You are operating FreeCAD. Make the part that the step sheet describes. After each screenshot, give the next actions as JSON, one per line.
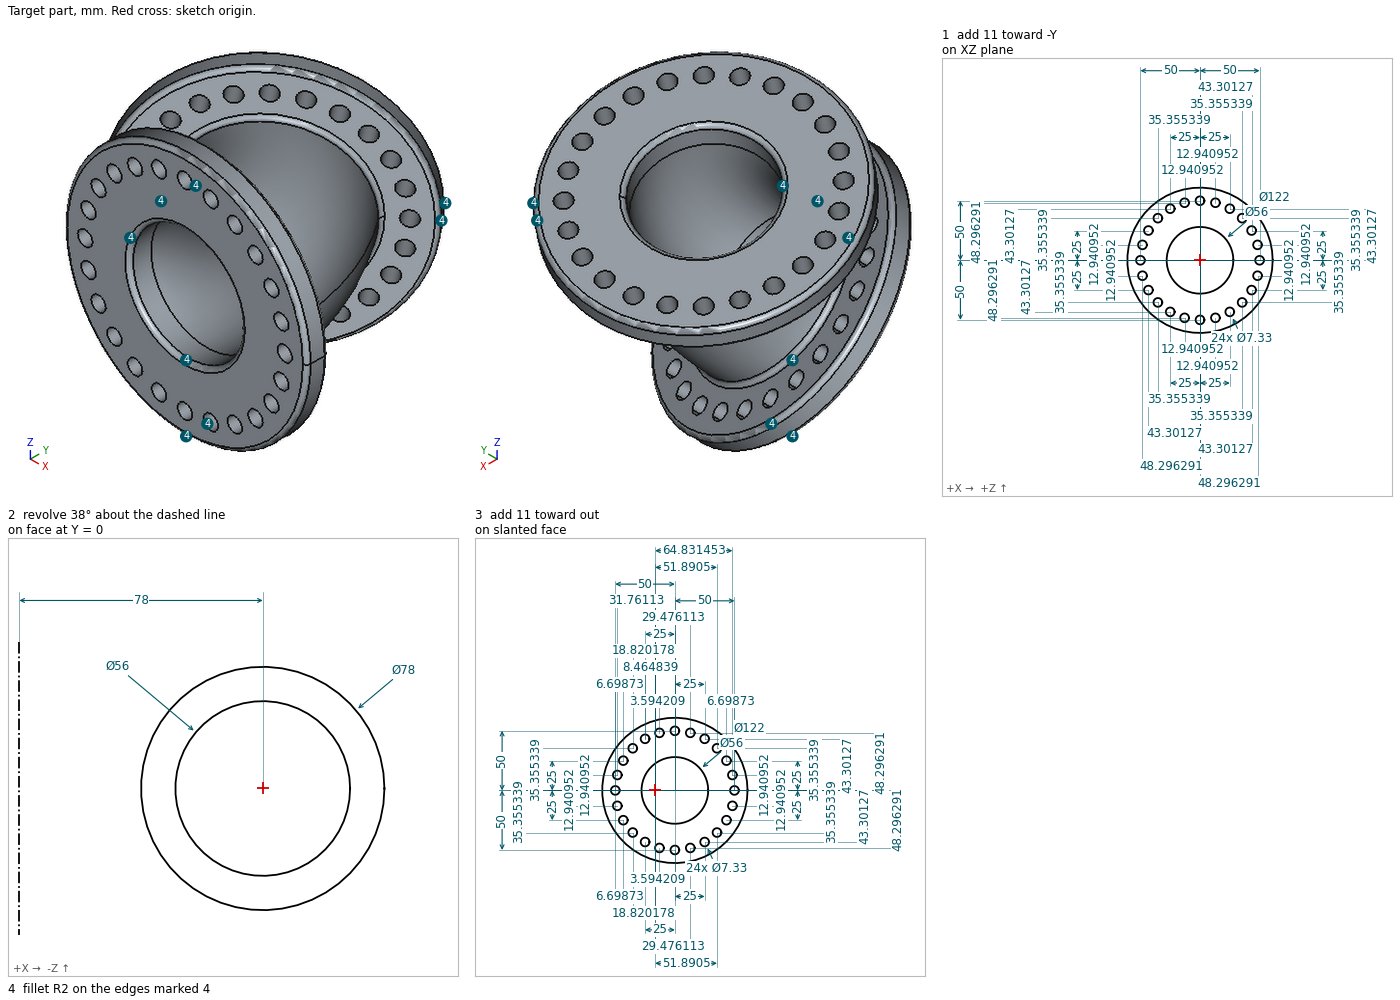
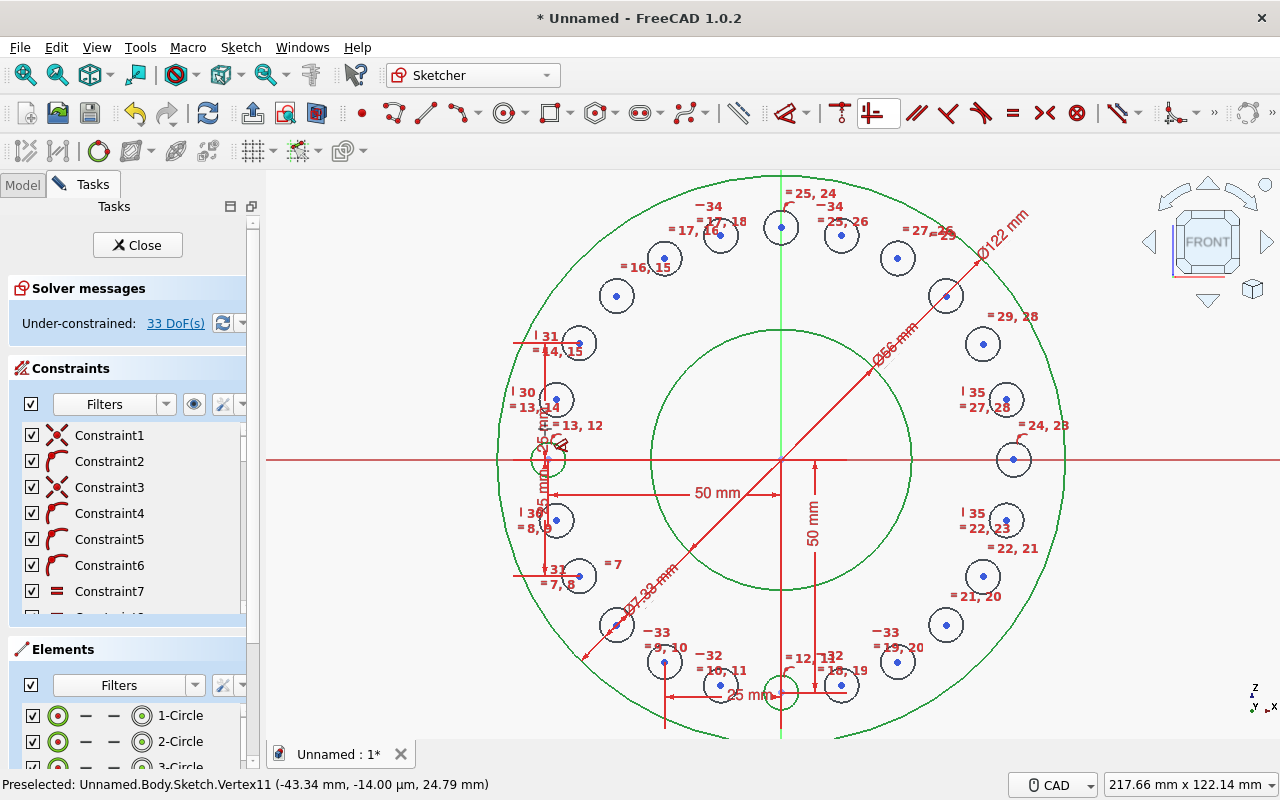
{"action": "left_click", "coordinate": [665, 259]}
{"action": "left_click", "coordinate": [750, 225]}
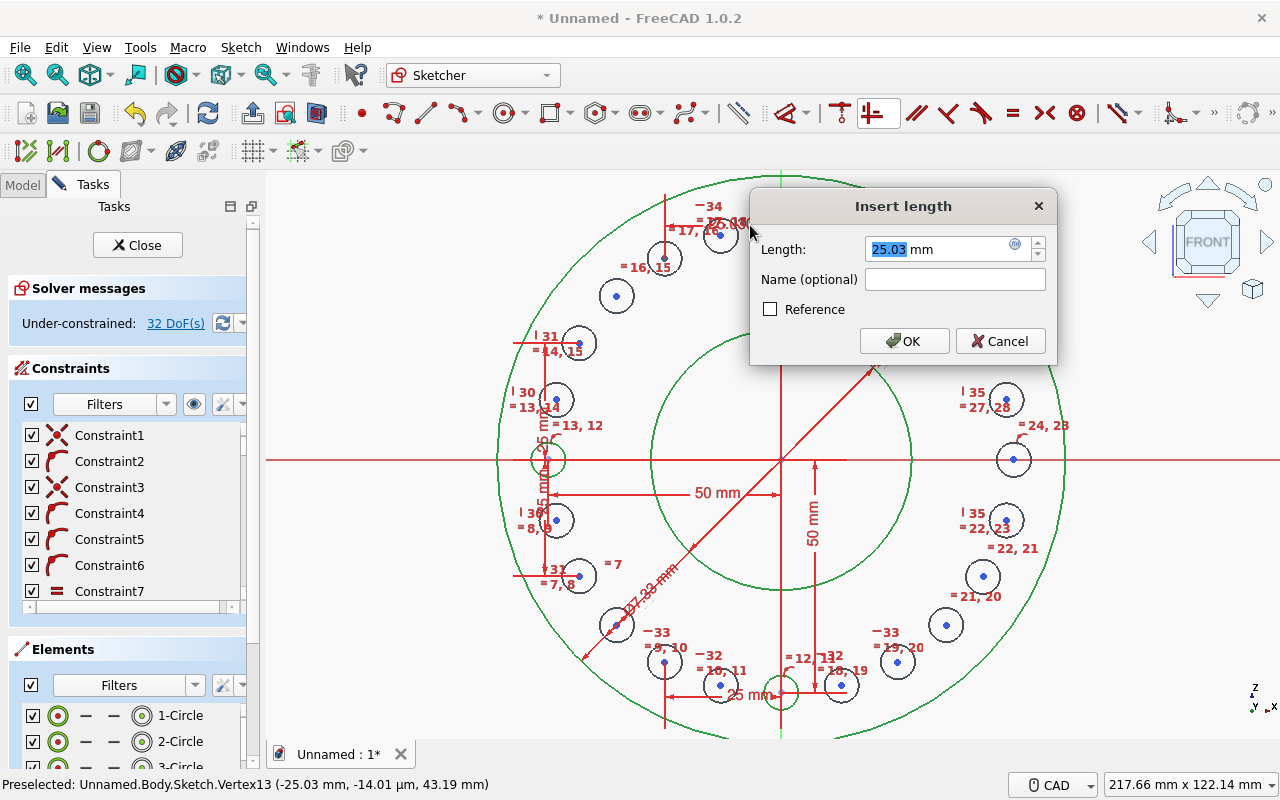
{"action": "type", "text": "25"}
{"action": "key", "text": "Return"}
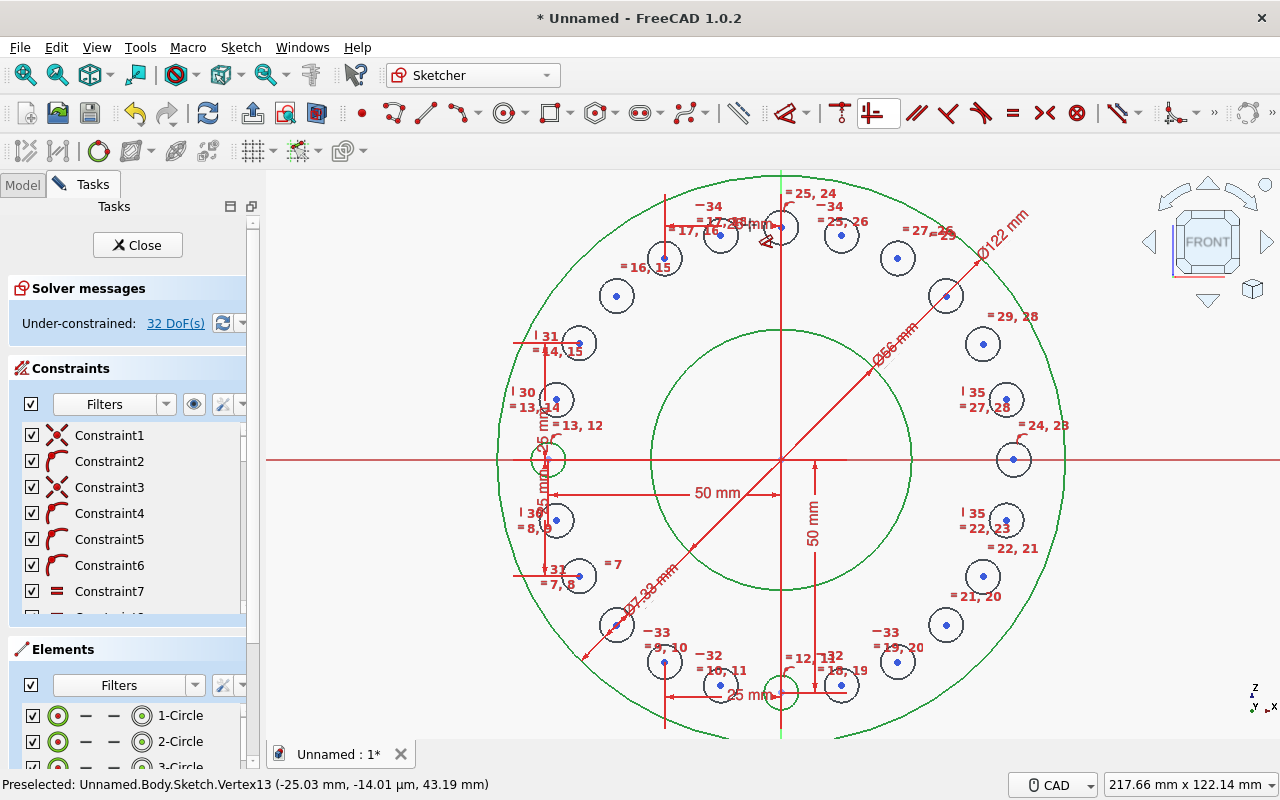
{"action": "left_click", "coordinate": [898, 662]}
{"action": "left_click", "coordinate": [880, 696]}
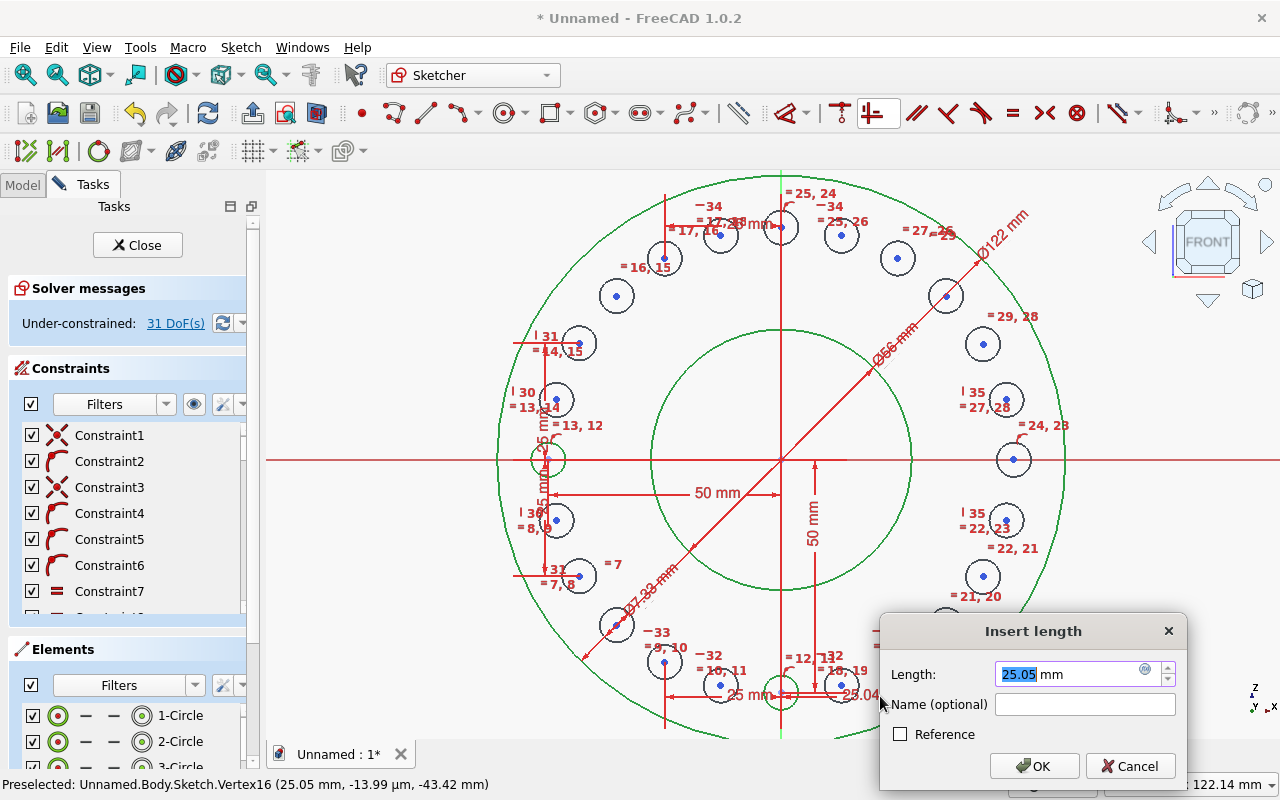
{"action": "type", "text": "25"}
{"action": "key", "text": "Return"}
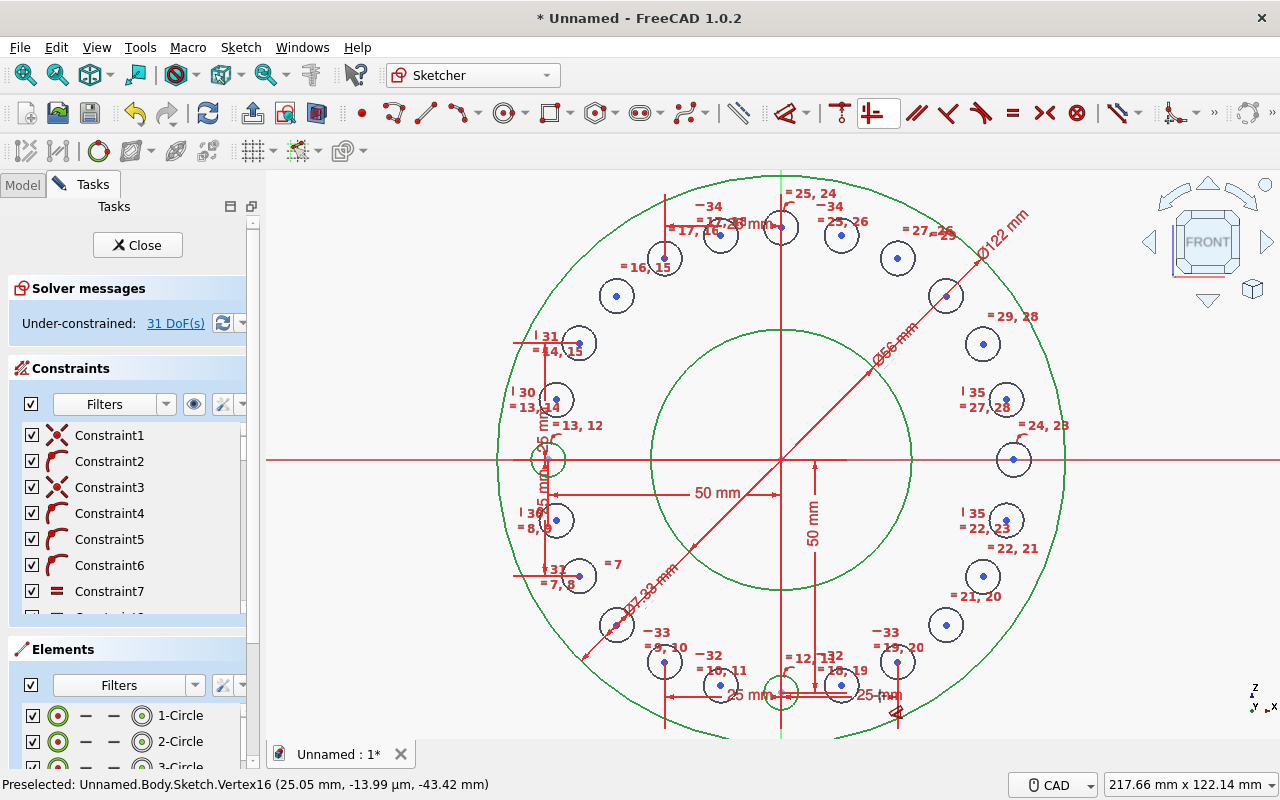
{"action": "left_click", "coordinate": [983, 577]}
{"action": "left_click", "coordinate": [1017, 491]}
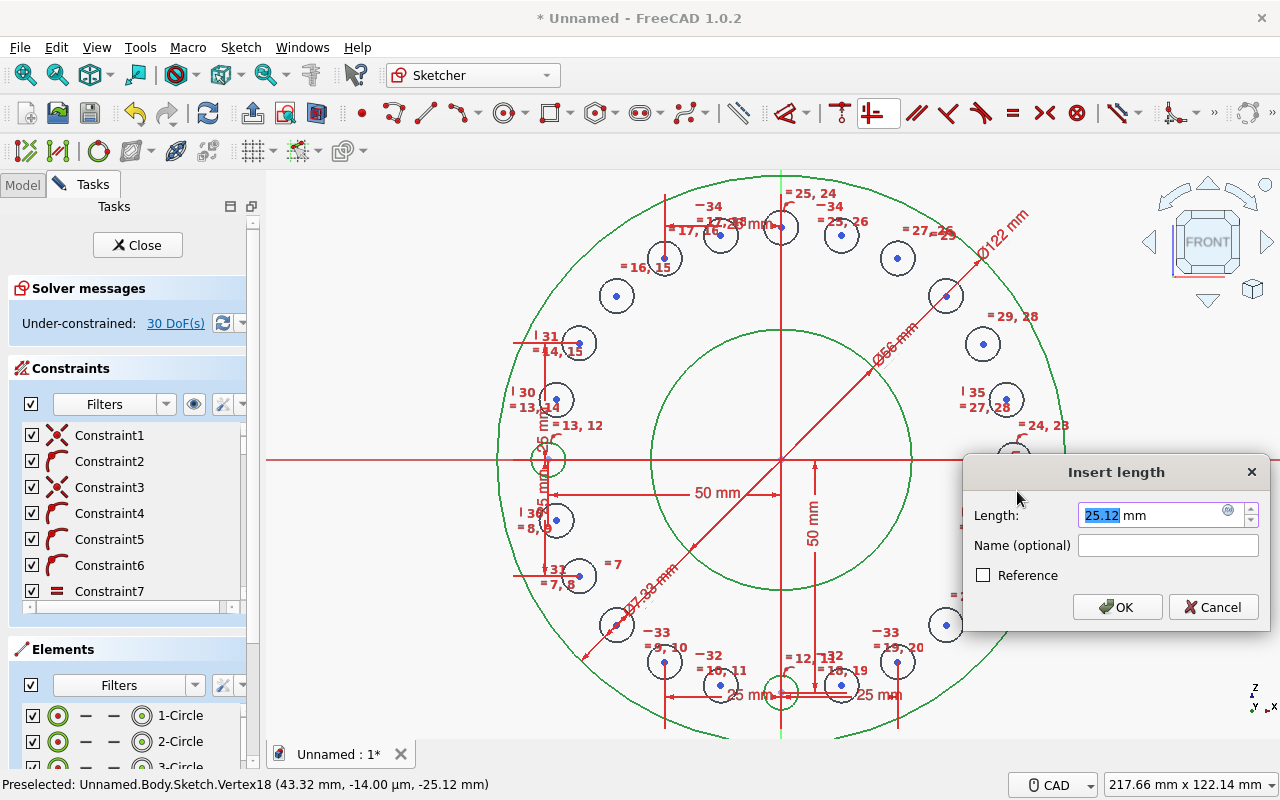
{"action": "type", "text": "25"}
{"action": "key", "text": "Return"}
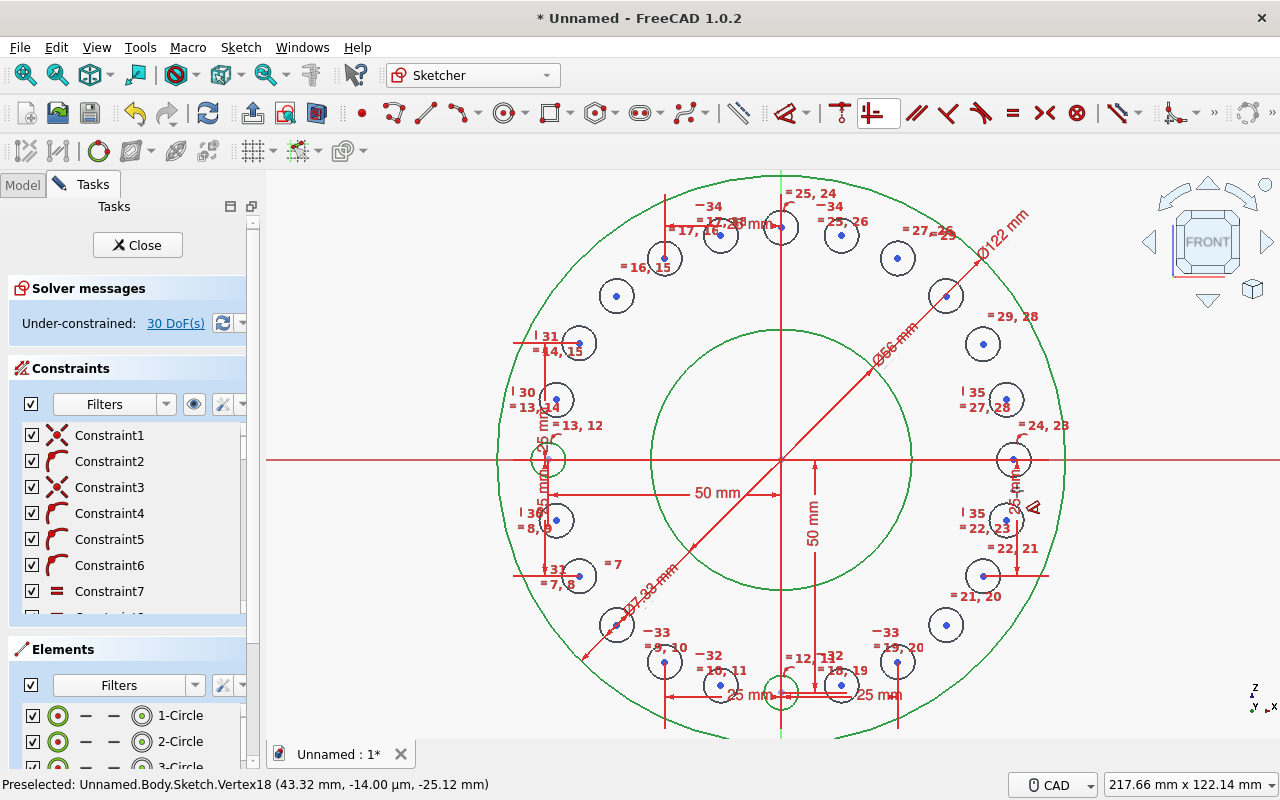
{"action": "left_click", "coordinate": [1014, 460]}
{"action": "left_click", "coordinate": [844, 494]}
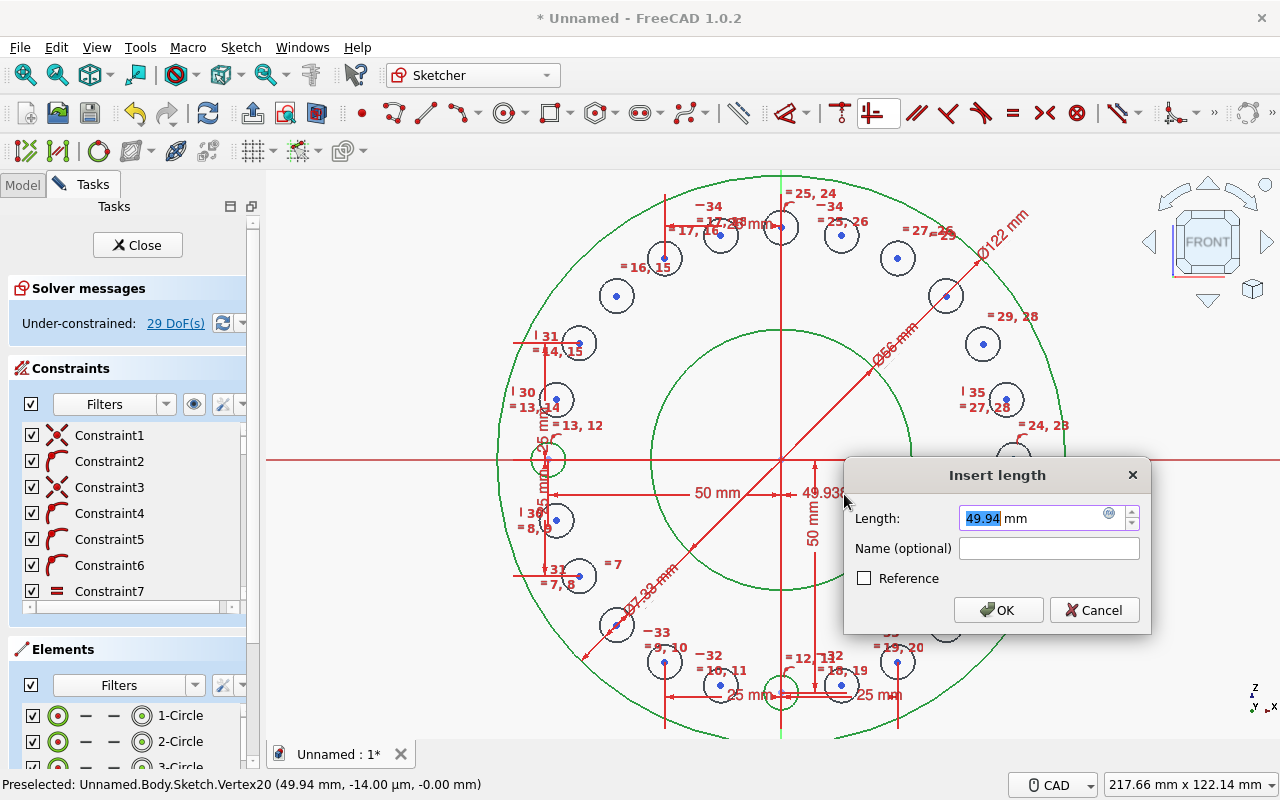
{"action": "type", "text": "50"}
{"action": "key", "text": "Return"}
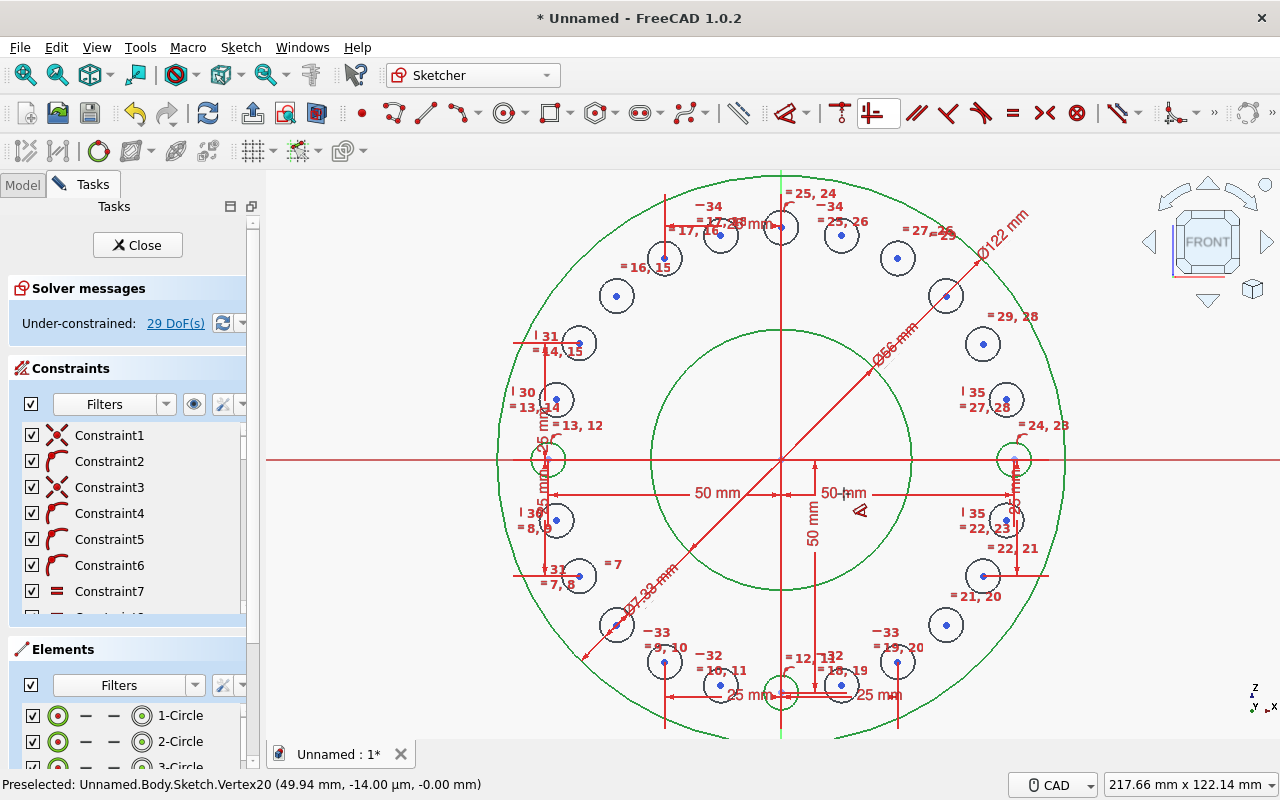
{"action": "left_click", "coordinate": [781, 228]}
{"action": "left_click", "coordinate": [815, 290]}